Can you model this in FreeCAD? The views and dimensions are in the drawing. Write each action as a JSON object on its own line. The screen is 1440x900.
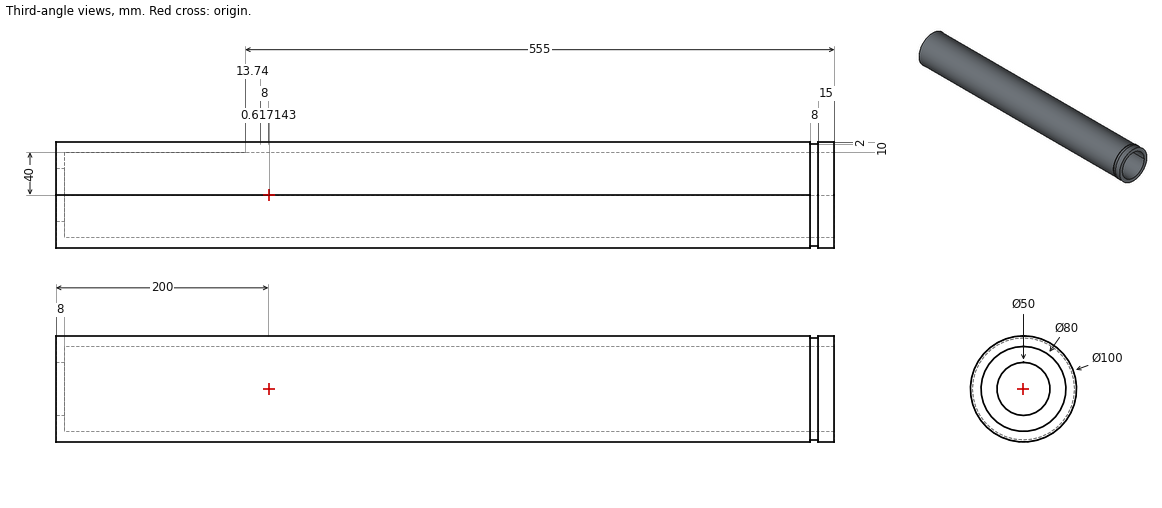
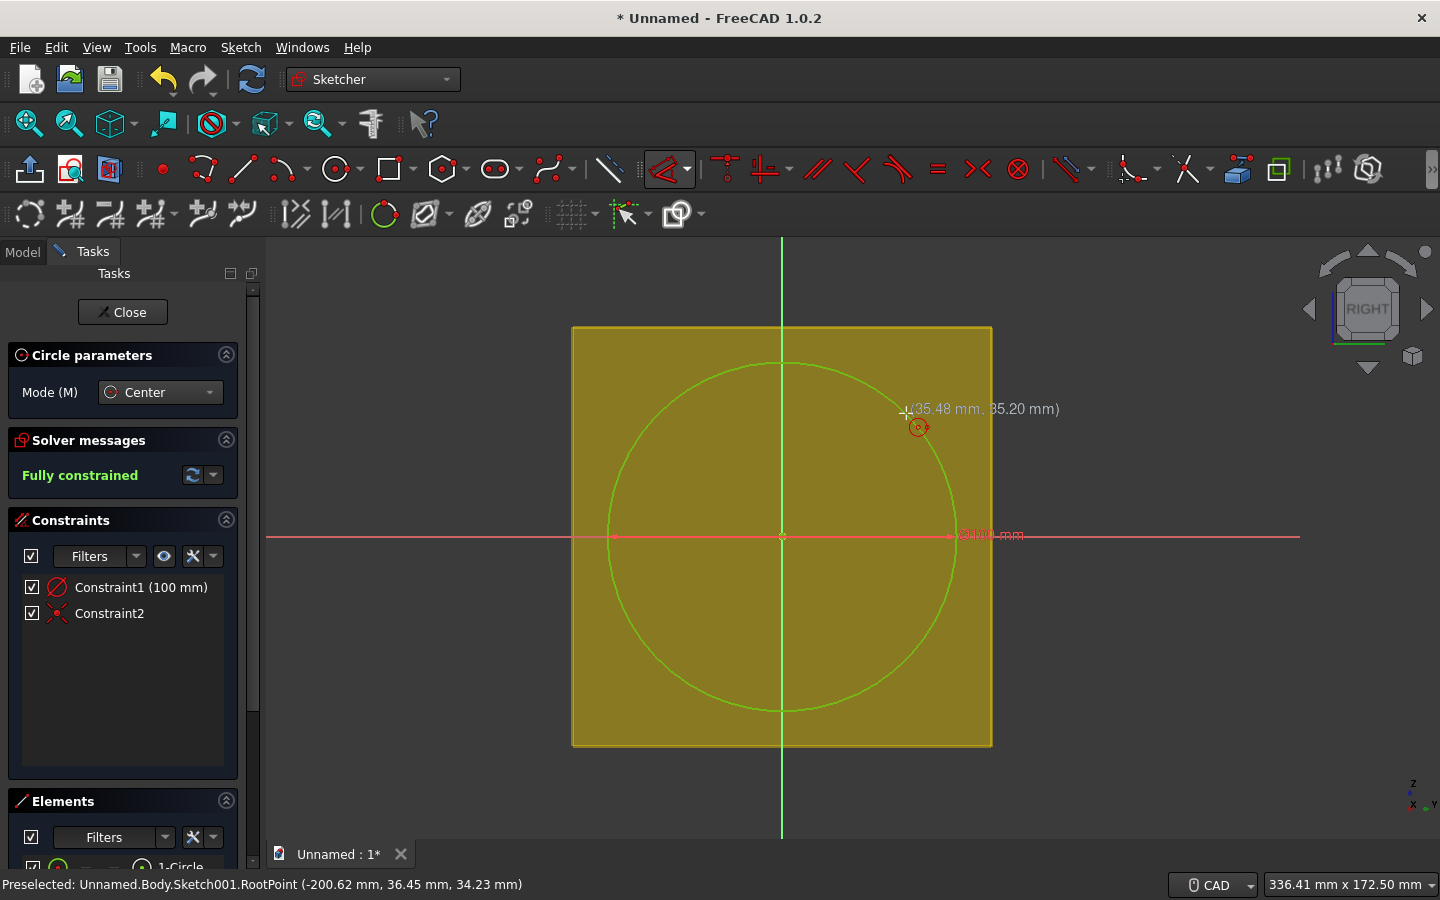
{"action": "left_click", "coordinate": [782, 537]}
{"action": "mouse_move", "coordinate": [881, 438]}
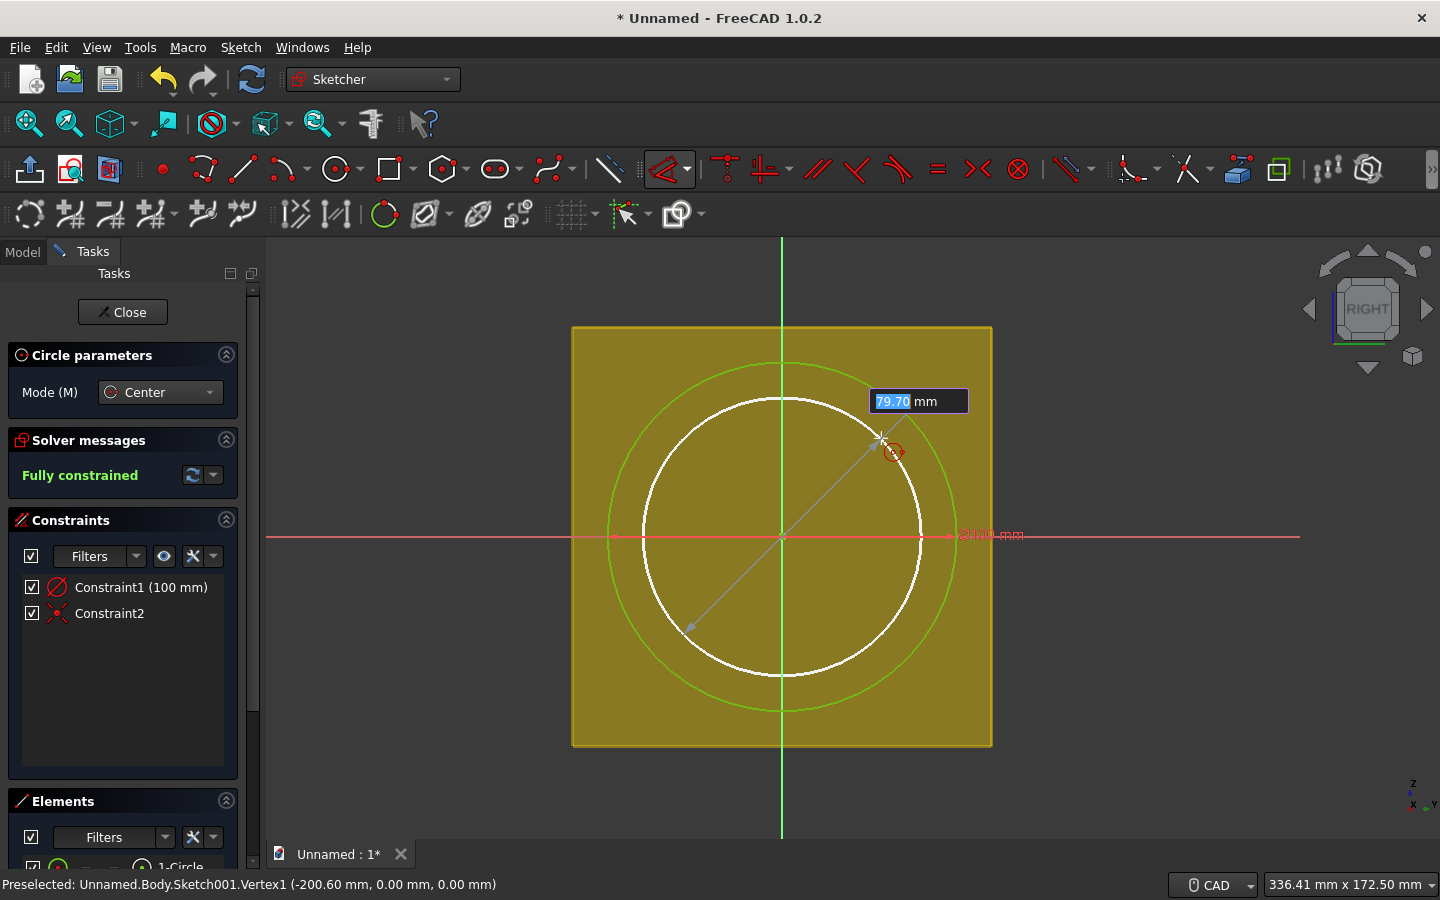
{"action": "type", "text": "80"}
{"action": "key", "text": "Return"}
{"action": "key", "text": "Escape"}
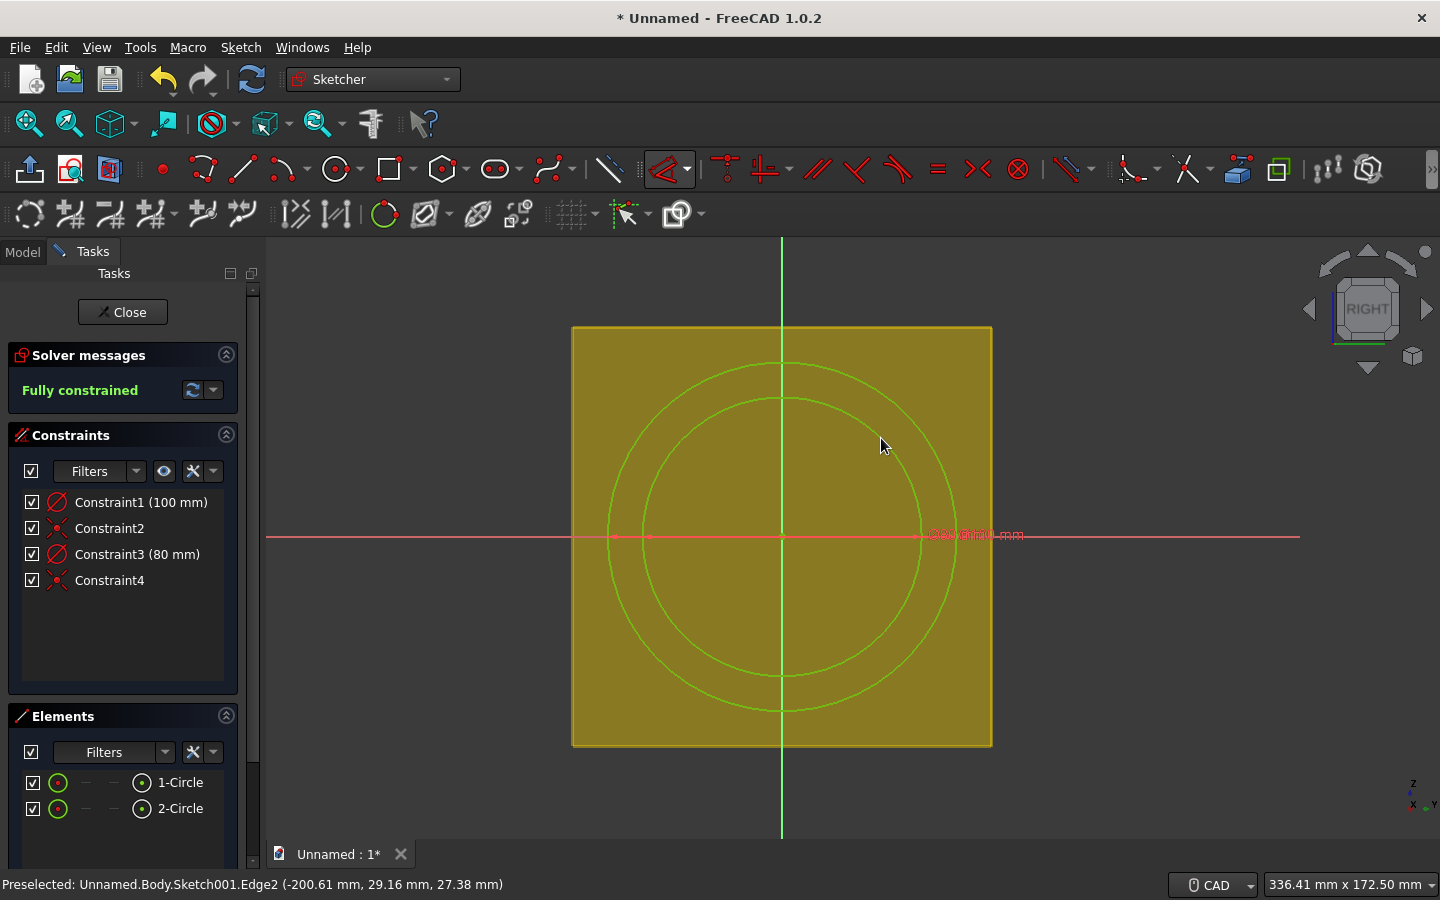
{"action": "left_click", "coordinate": [123, 312]}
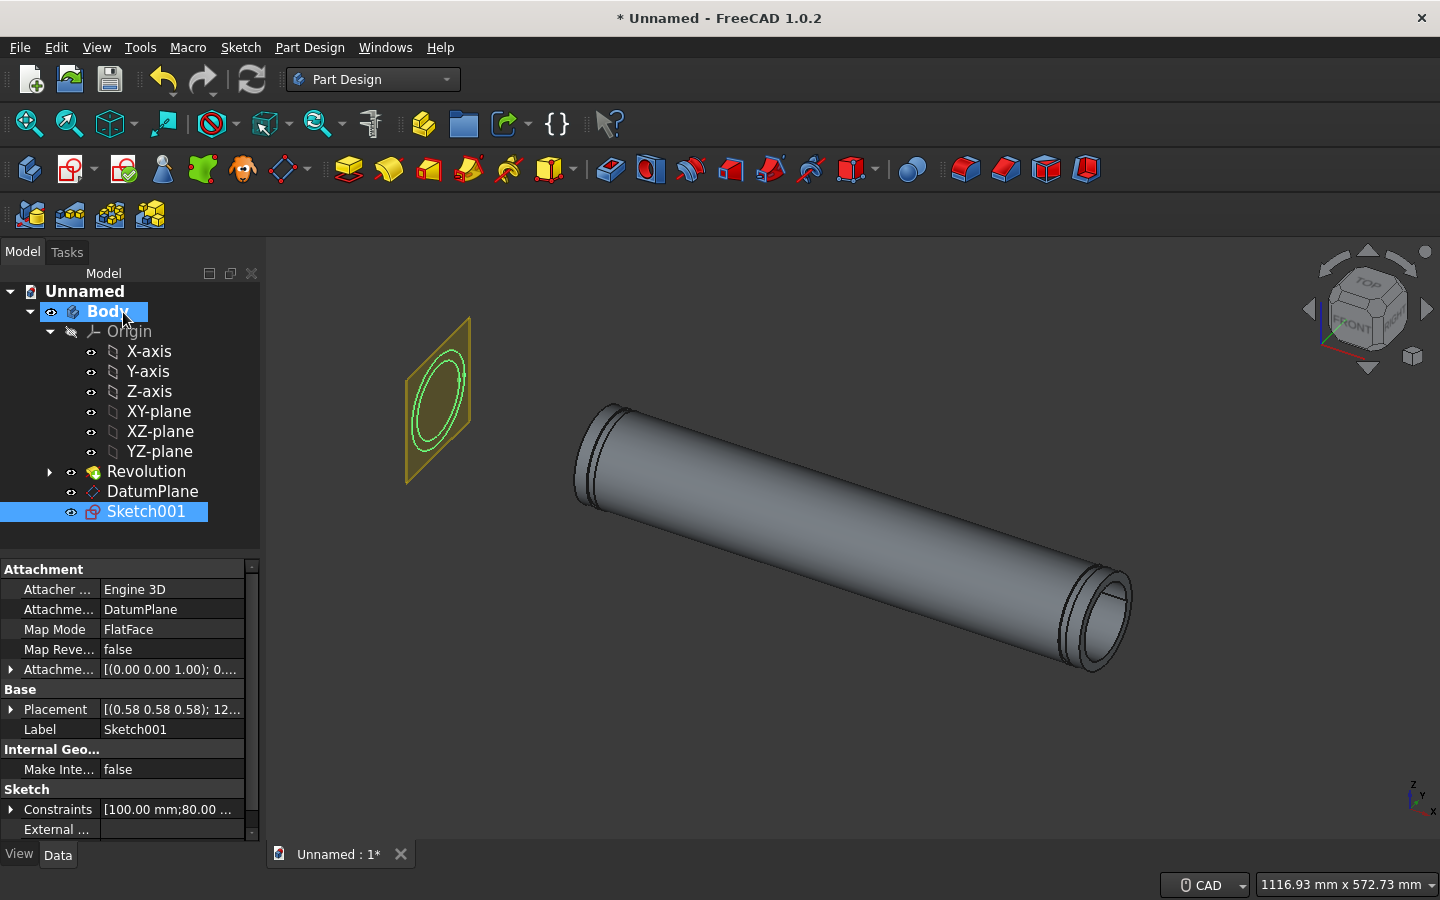
{"action": "left_click", "coordinate": [350, 170]}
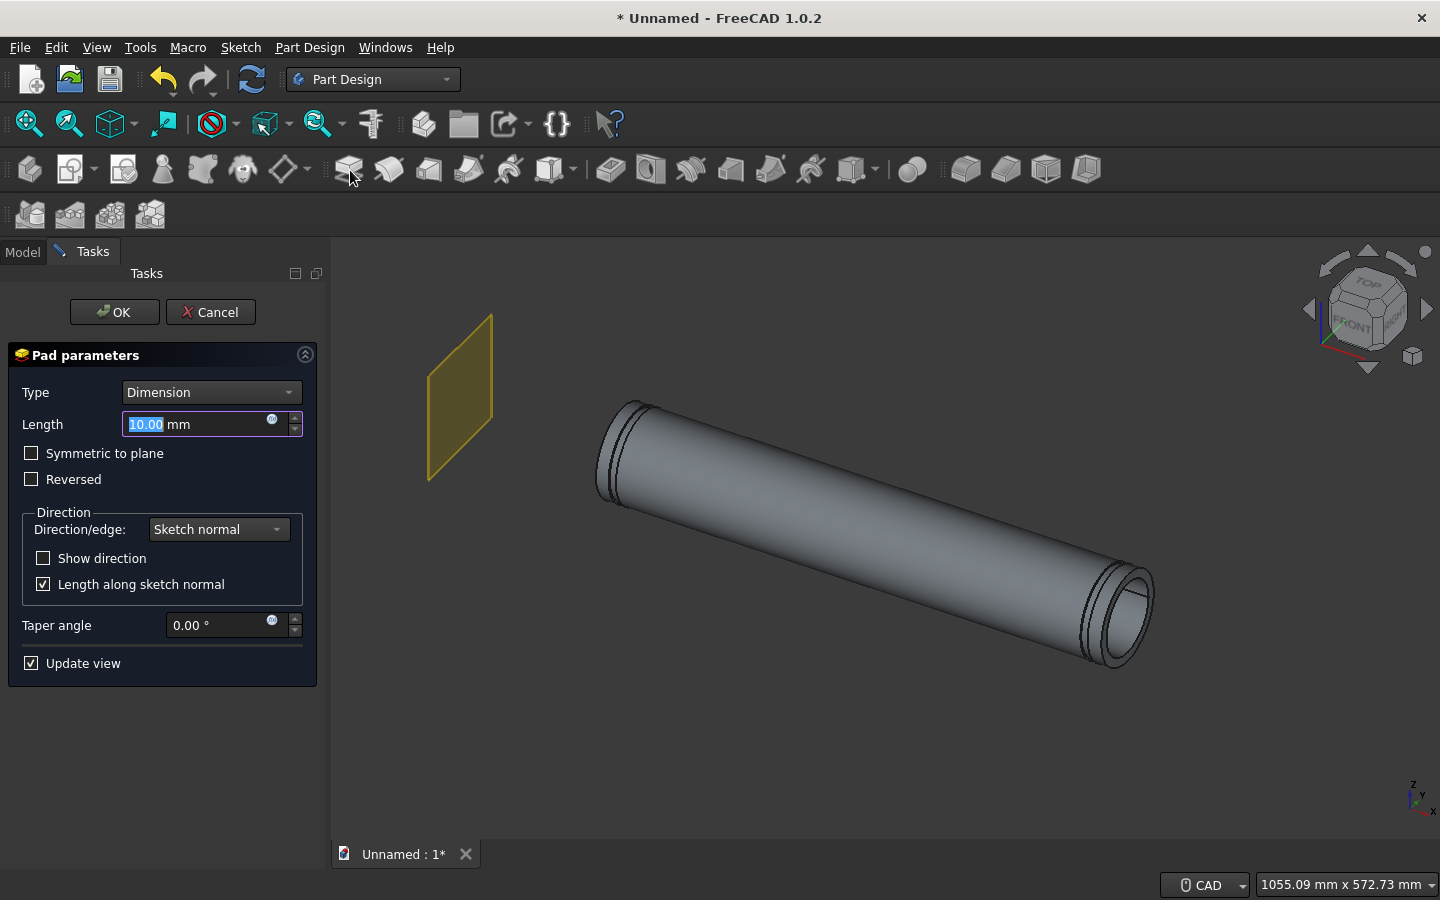
{"action": "type", "text": "200"}
{"action": "key", "text": "Tab"}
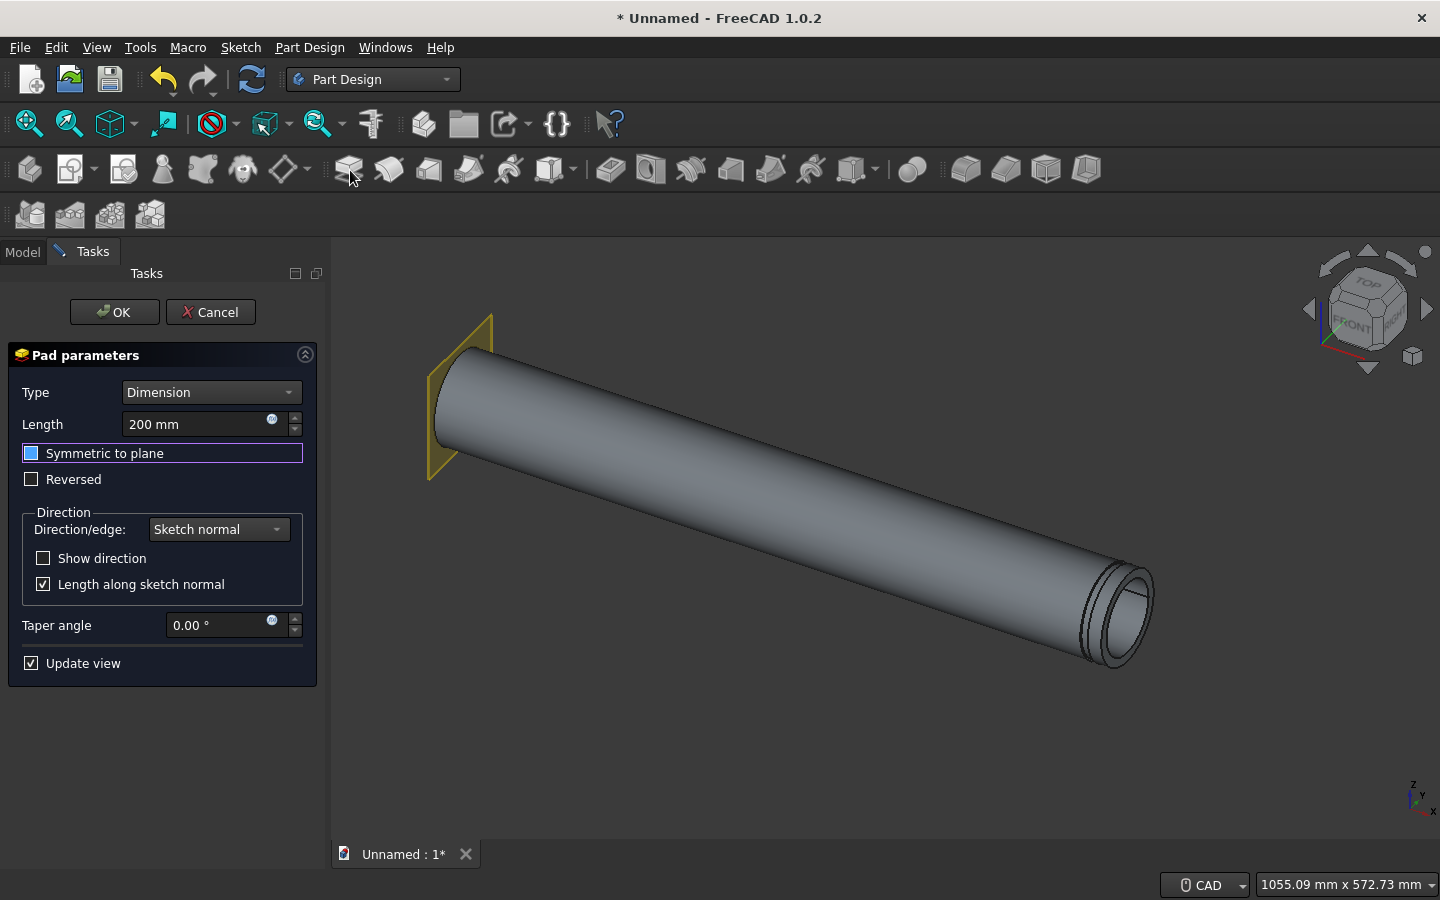
{"action": "left_click", "coordinate": [115, 312]}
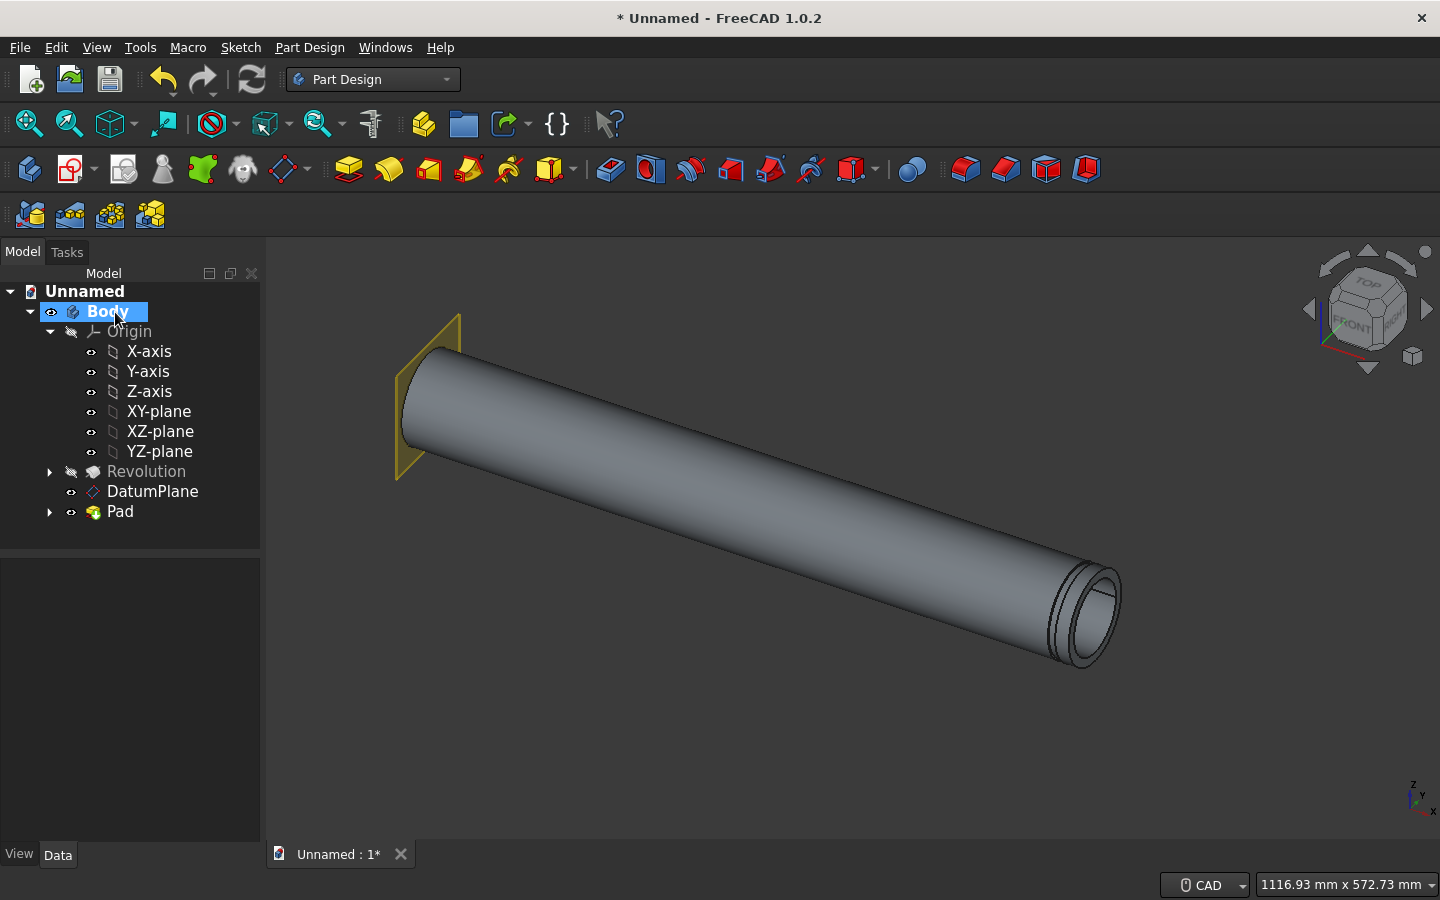
{"action": "left_click", "coordinate": [116, 492]}
{"action": "key", "text": "space"}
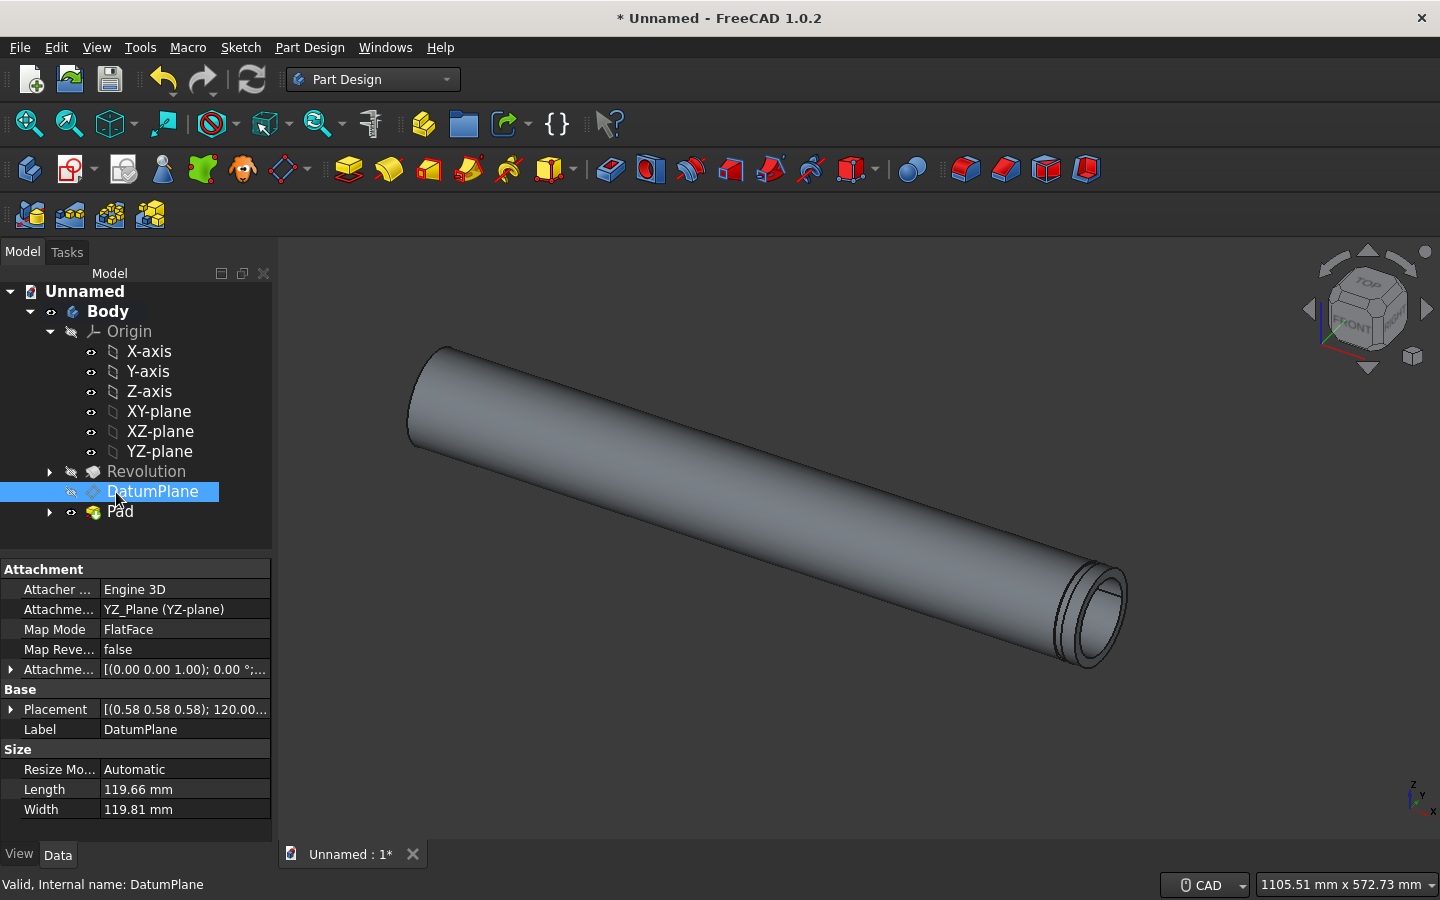
{"action": "left_click", "coordinate": [136, 452]}